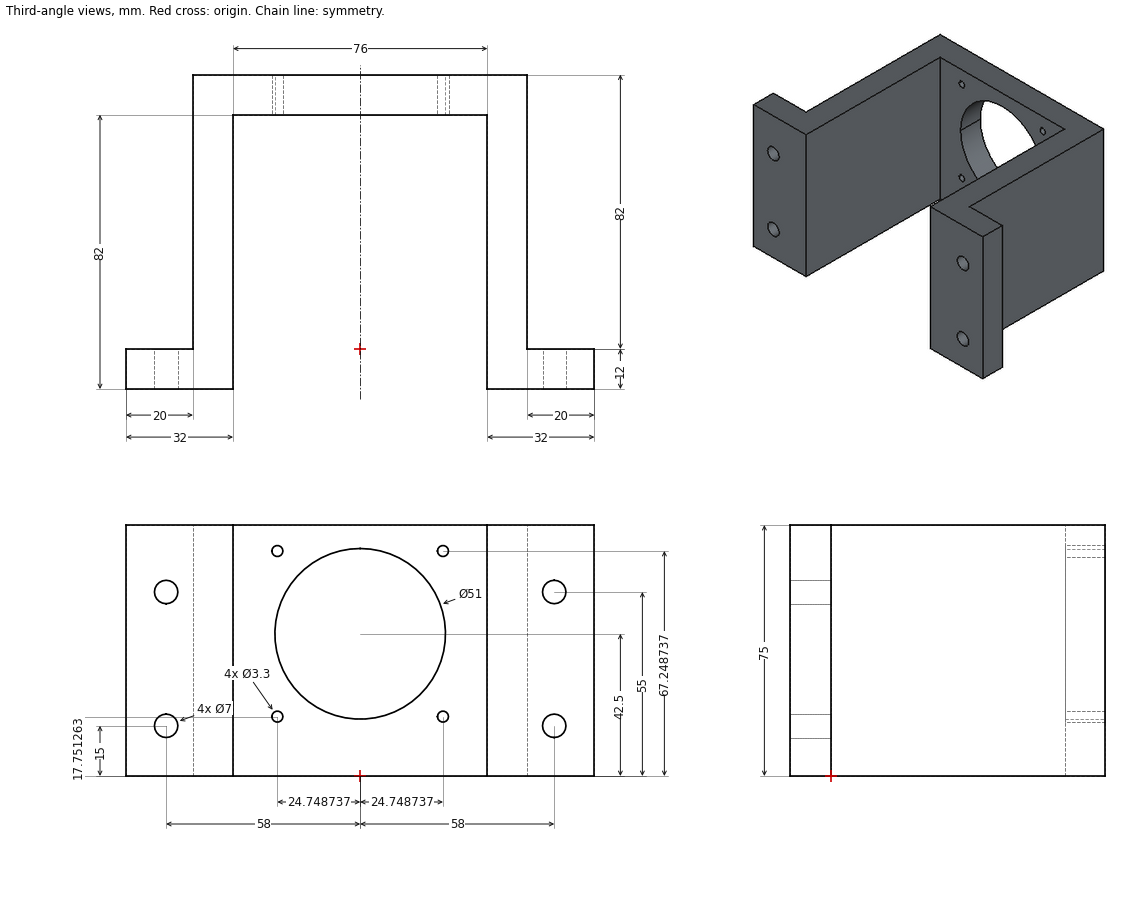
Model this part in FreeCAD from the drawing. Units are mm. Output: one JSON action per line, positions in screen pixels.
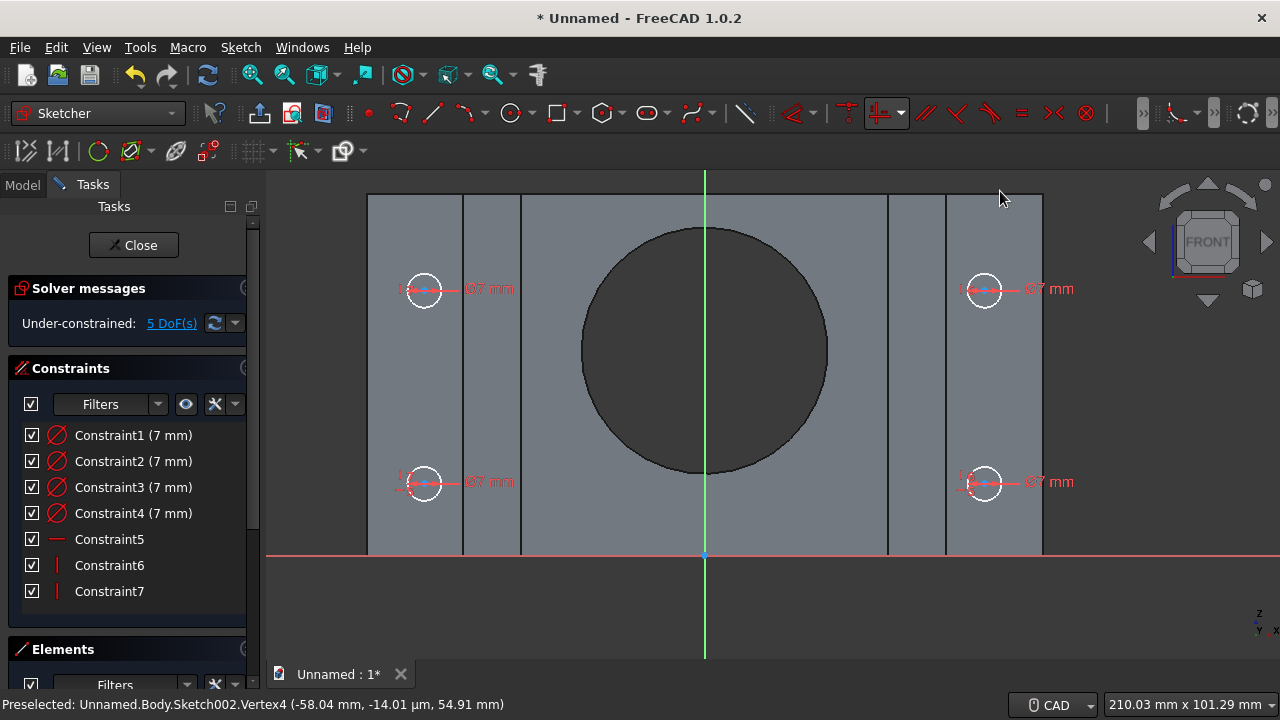
{"action": "left_click", "coordinate": [985, 291]}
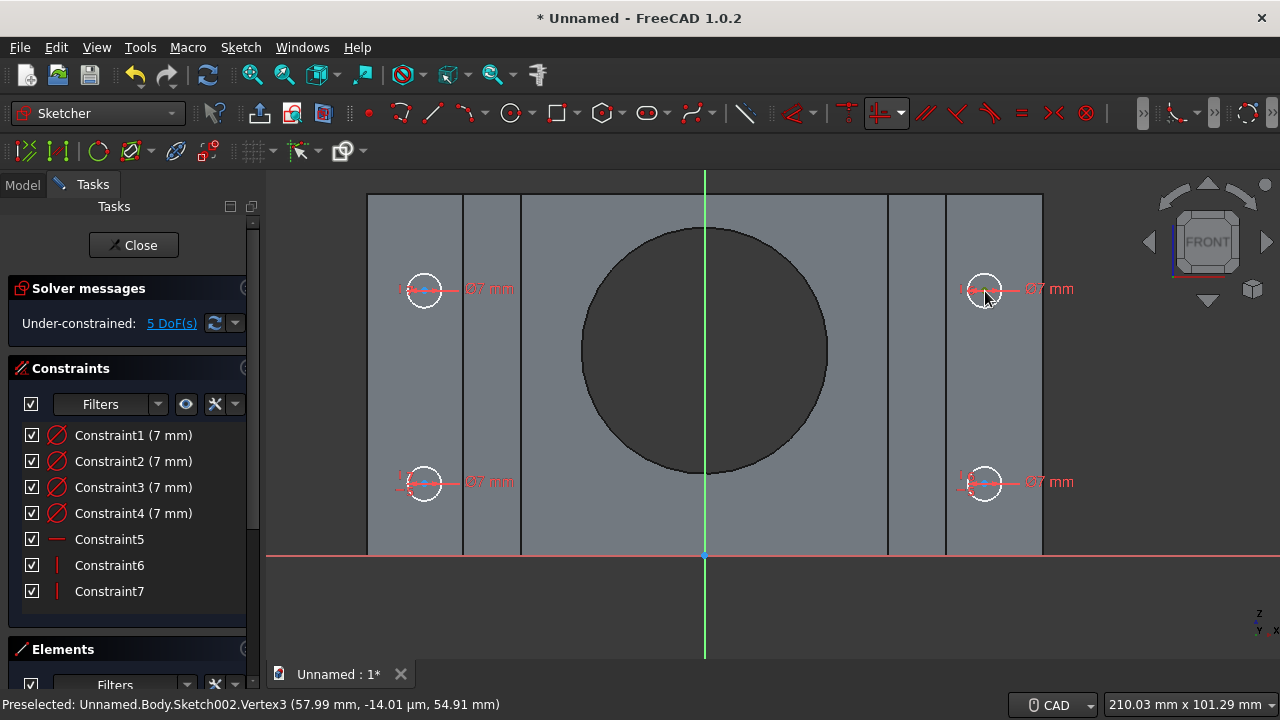
{"action": "left_click", "coordinate": [424, 291]}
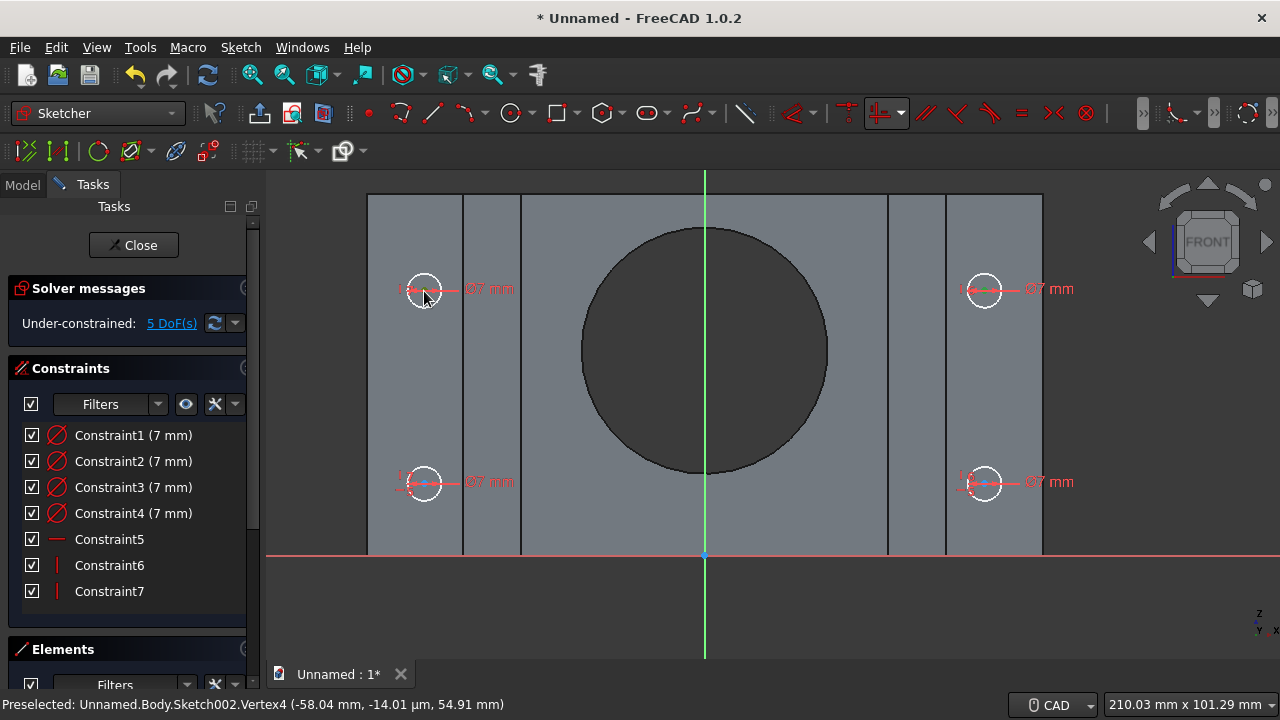
{"action": "left_click", "coordinate": [904, 114]}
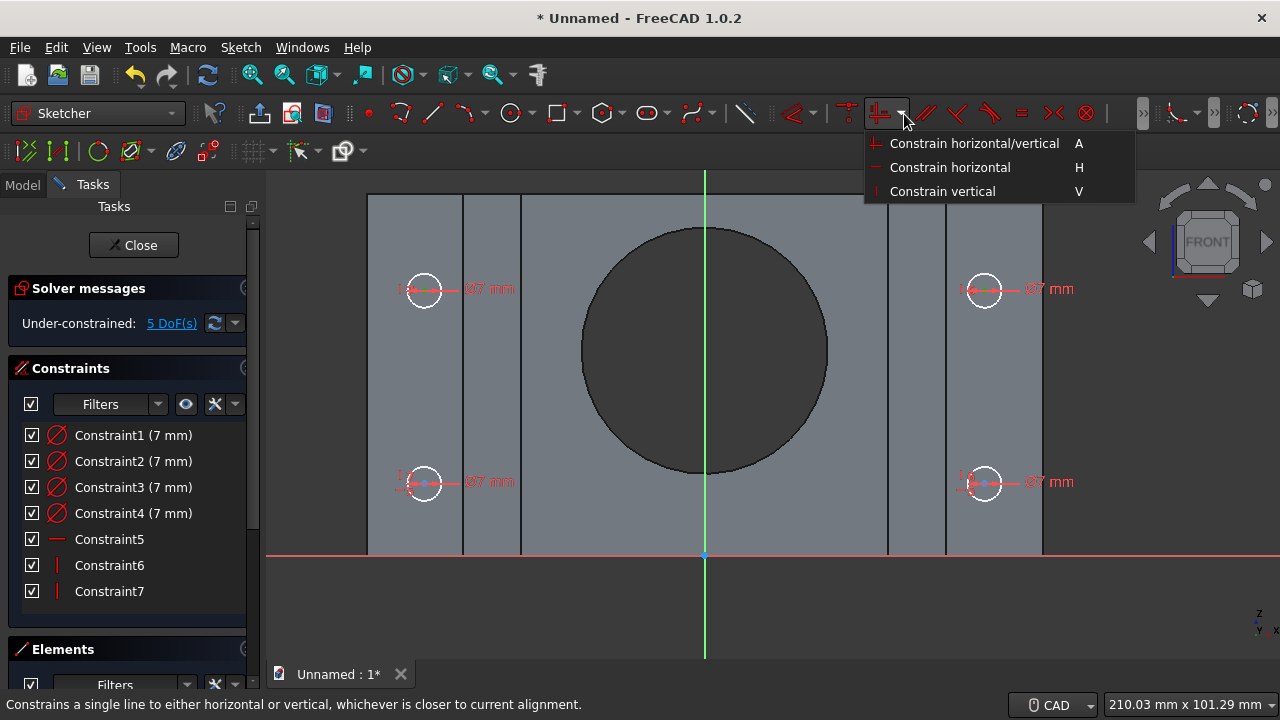
{"action": "left_click", "coordinate": [1000, 167]}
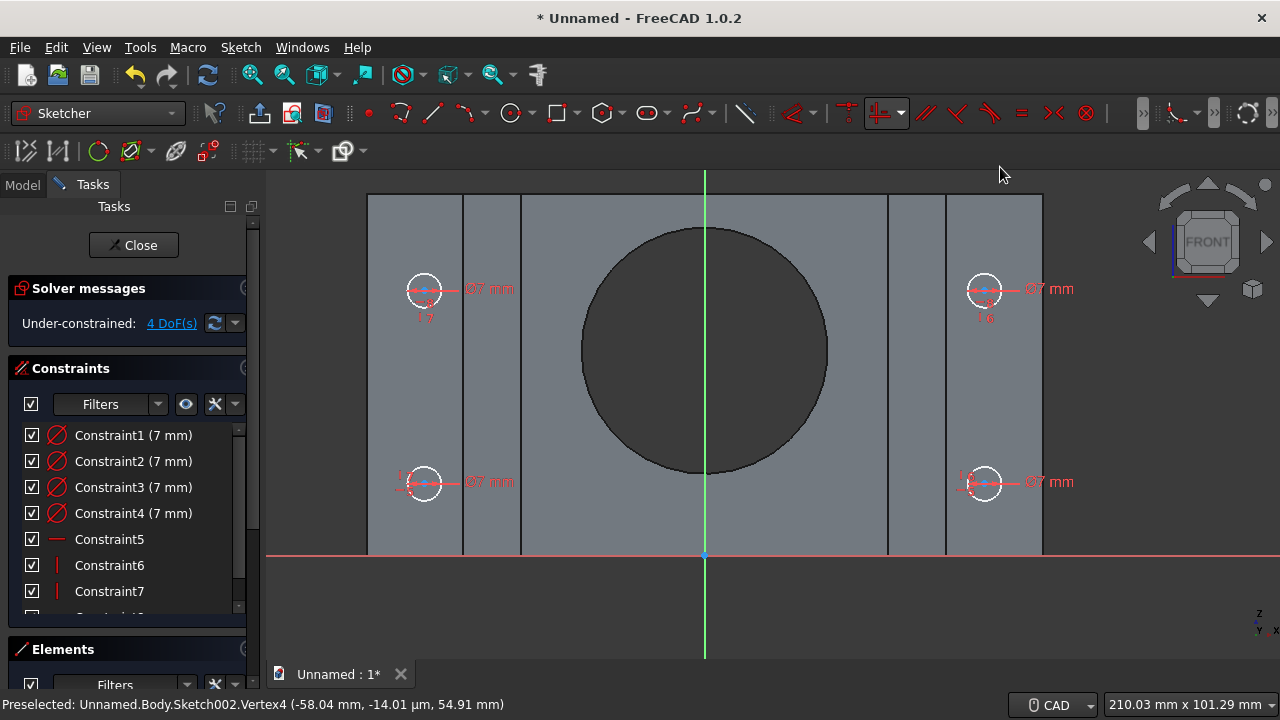
{"action": "left_click", "coordinate": [792, 114]}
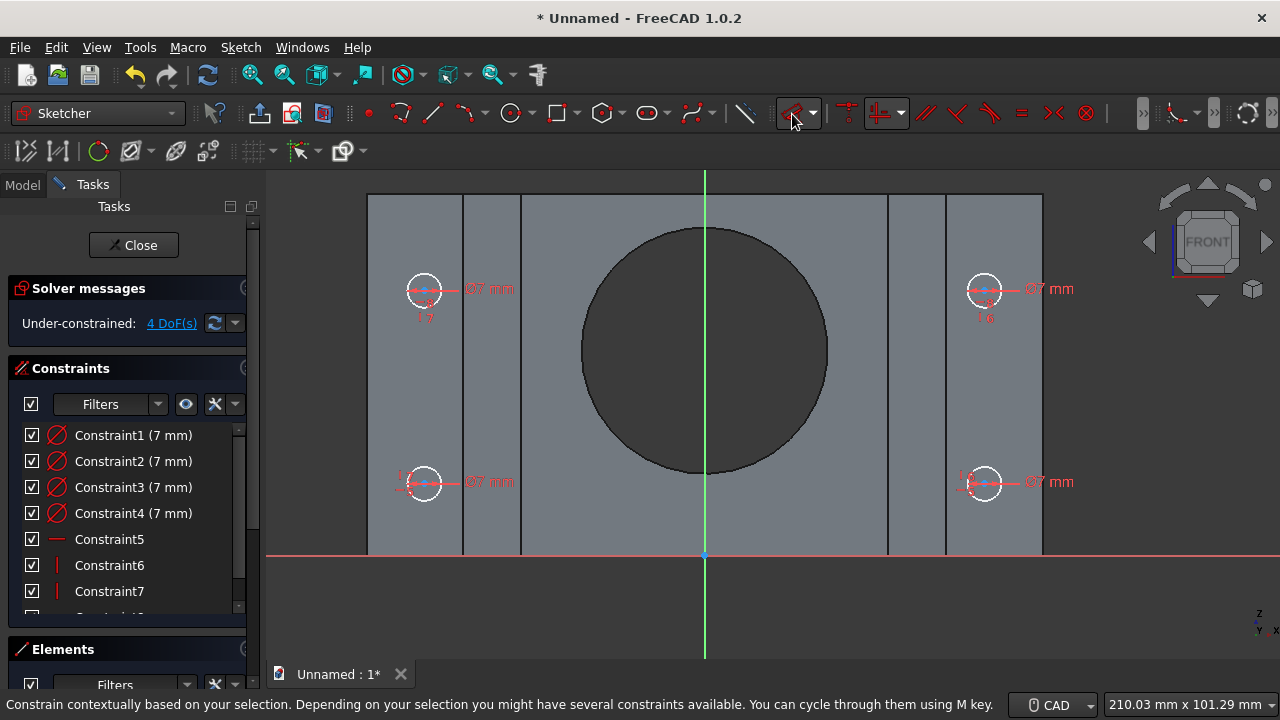
{"action": "left_click", "coordinate": [424, 484]}
{"action": "left_click", "coordinate": [564, 590]}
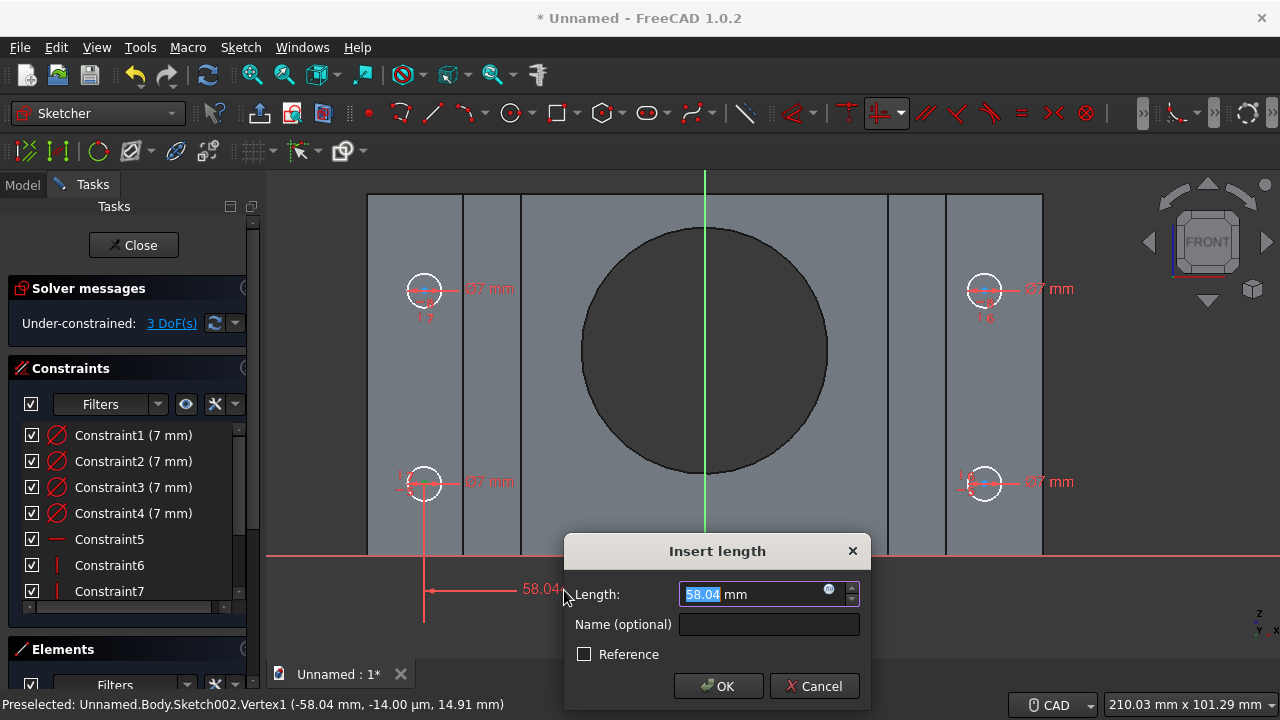
{"action": "type", "text": "58"}
{"action": "key", "text": "Return"}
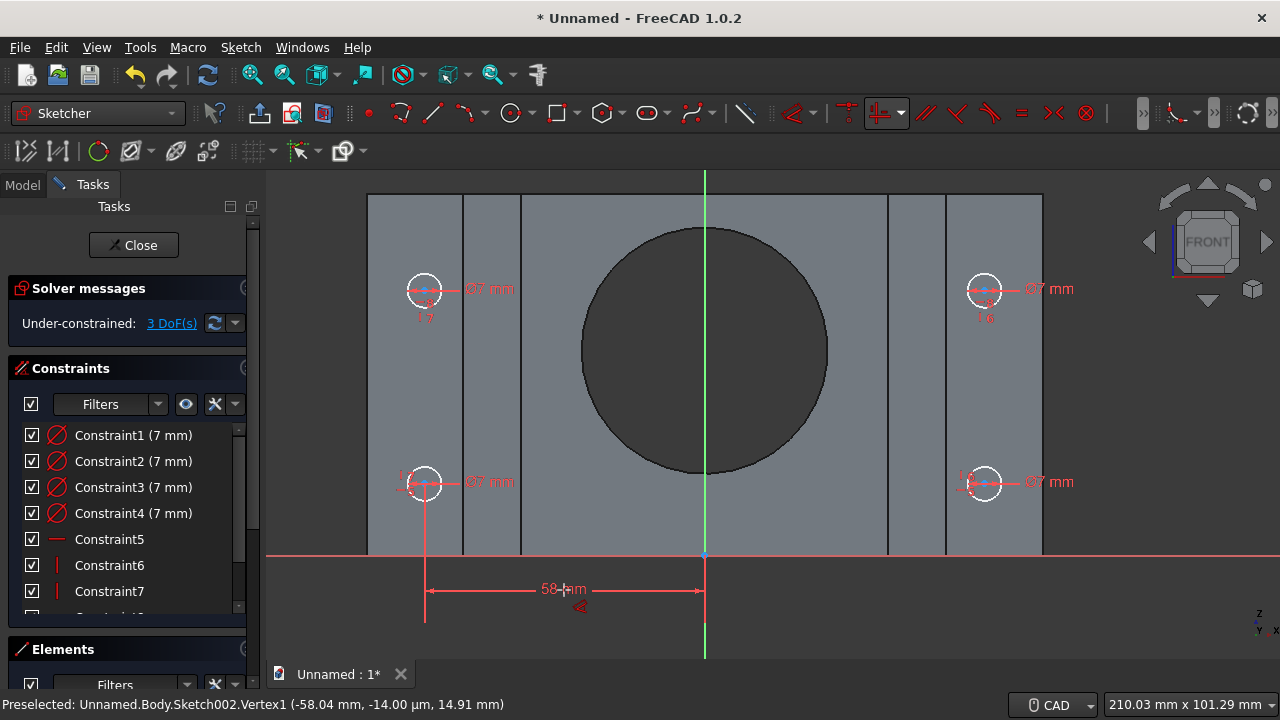
{"action": "left_click", "coordinate": [425, 484]}
{"action": "left_click", "coordinate": [391, 520]}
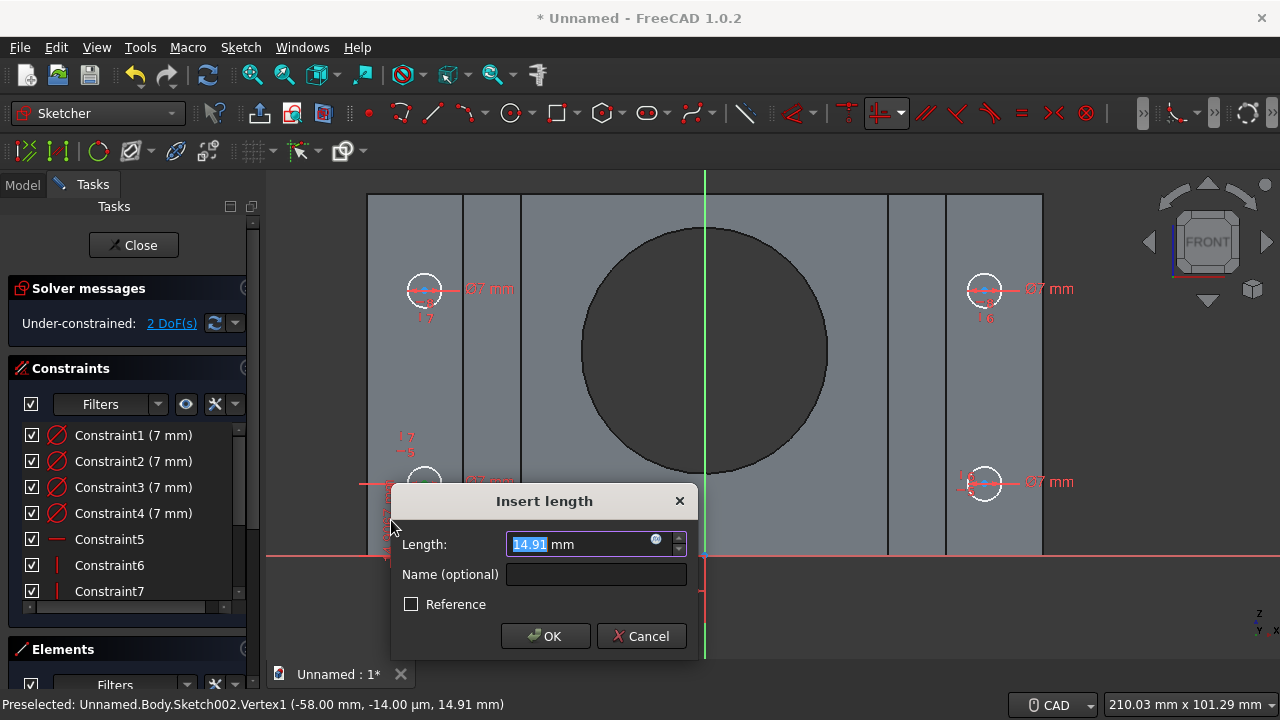
{"action": "type", "text": "15"}
{"action": "key", "text": "Return"}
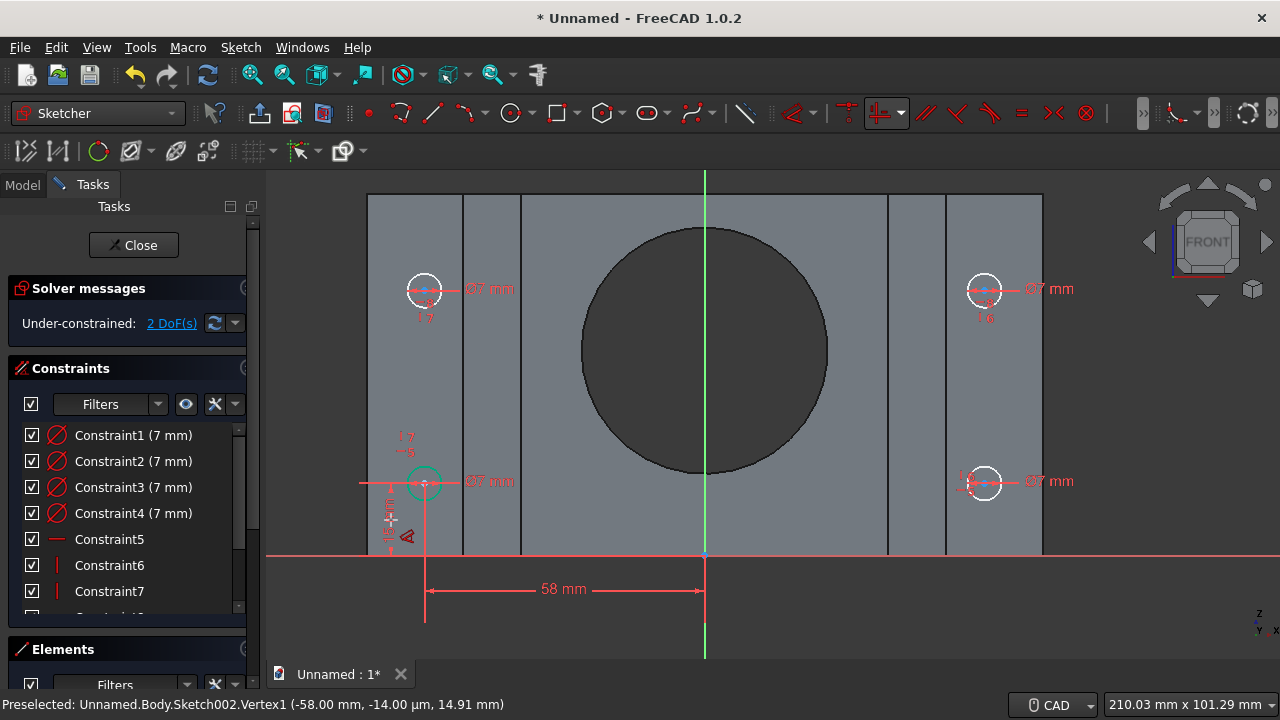
{"action": "left_click", "coordinate": [985, 483]}
{"action": "left_click", "coordinate": [845, 590]}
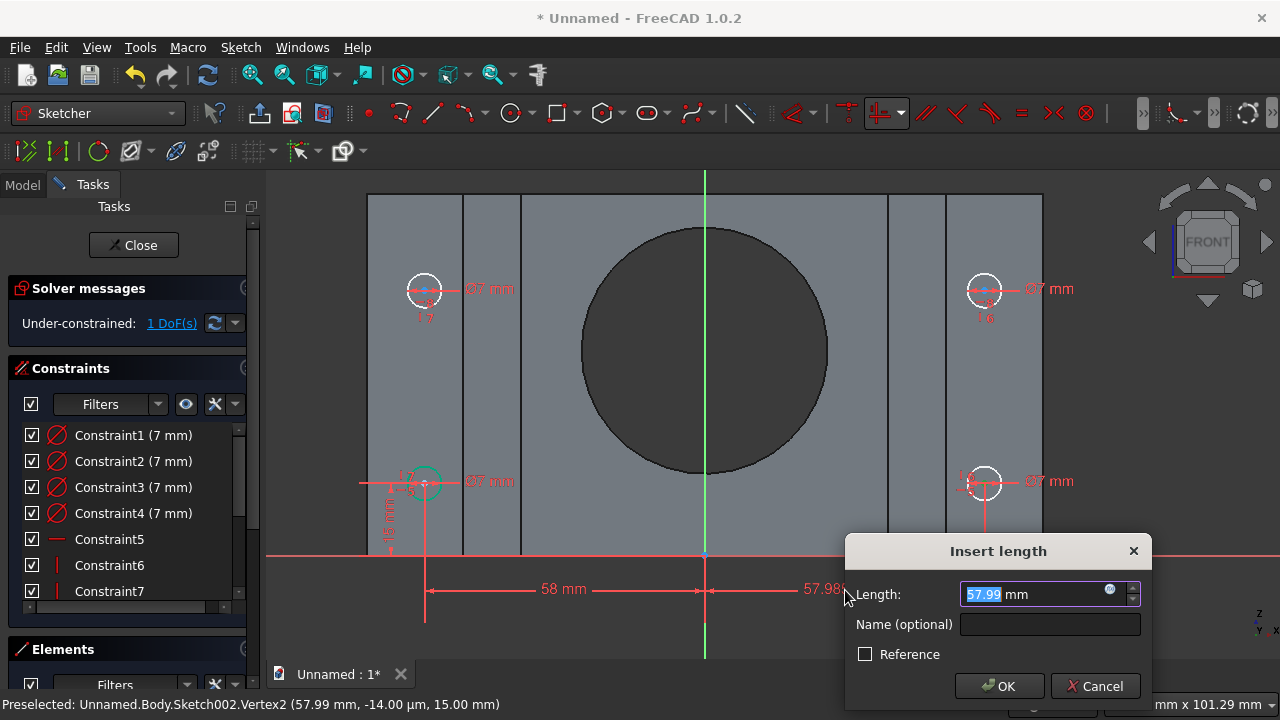
{"action": "type", "text": "58"}
{"action": "key", "text": "Return"}